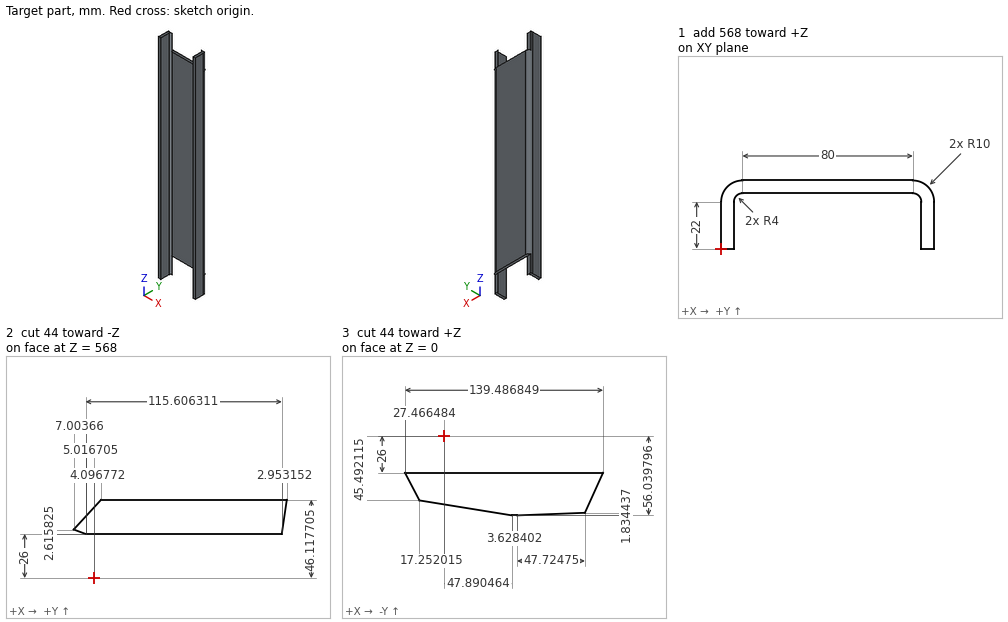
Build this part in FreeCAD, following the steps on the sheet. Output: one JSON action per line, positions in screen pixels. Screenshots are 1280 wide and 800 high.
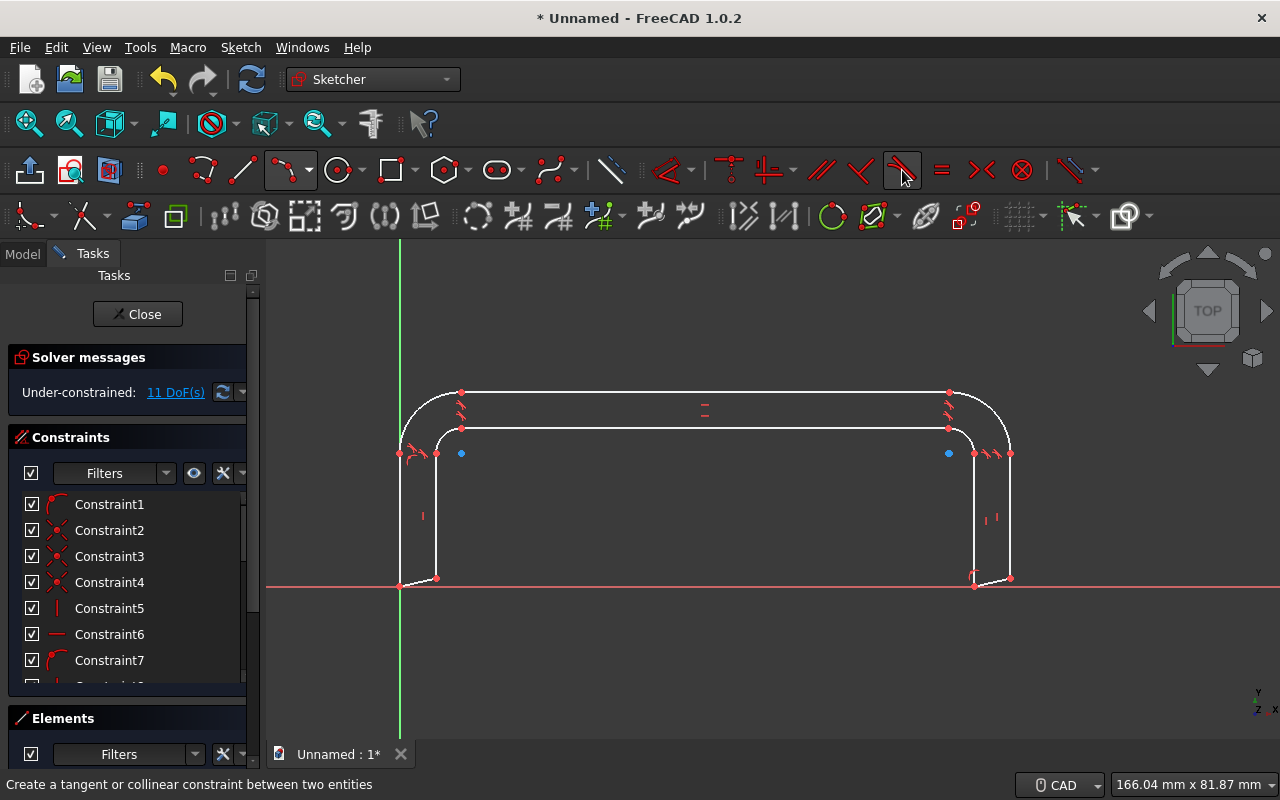
{"action": "scroll", "coordinate": [411, 584], "scroll_direction": "up", "scroll_amount": 2}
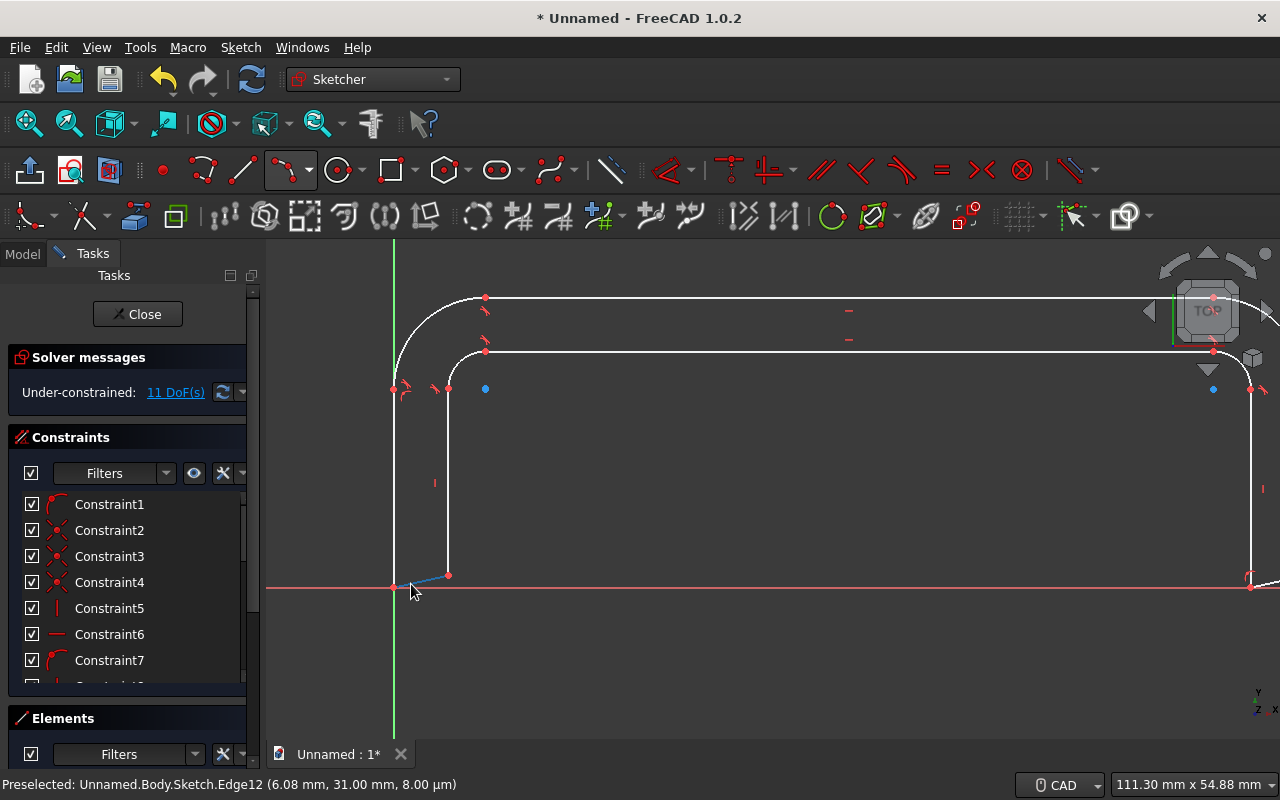
{"action": "left_click", "coordinate": [410, 584]}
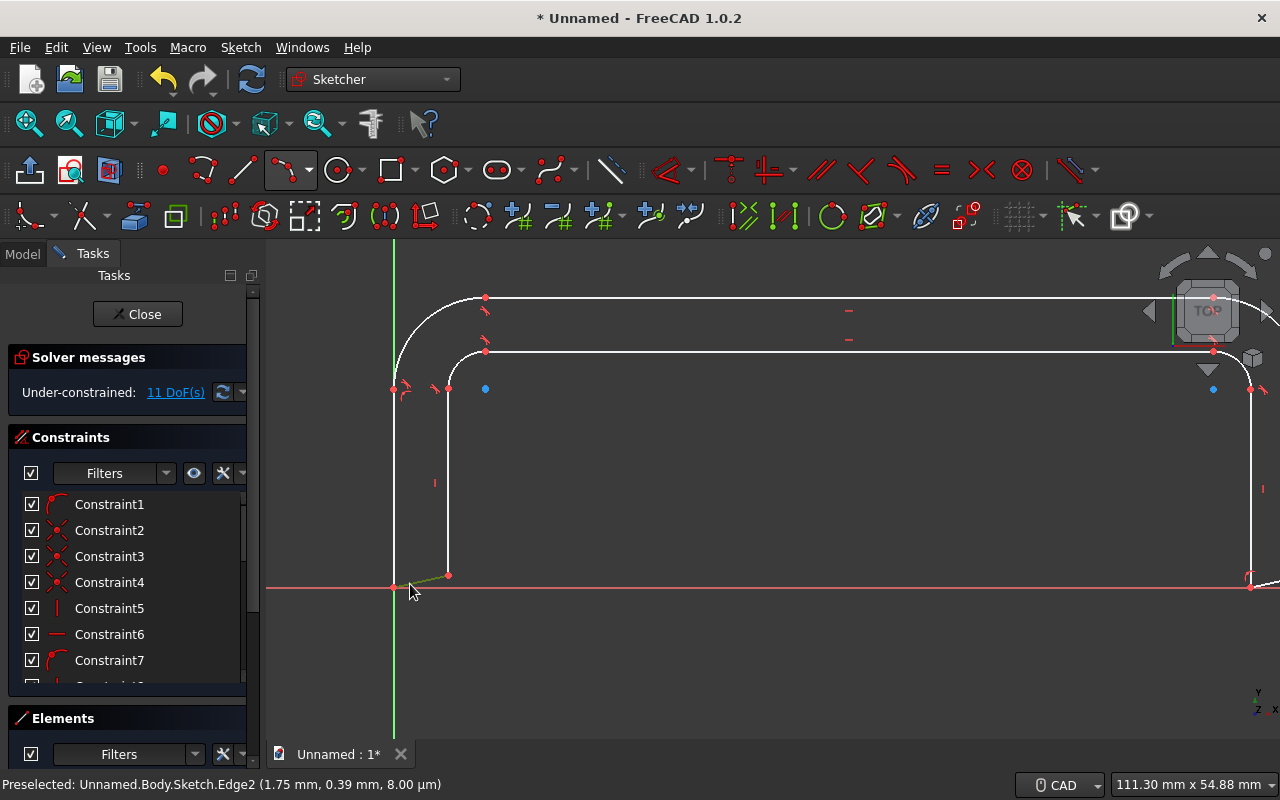
{"action": "left_click", "coordinate": [796, 170]}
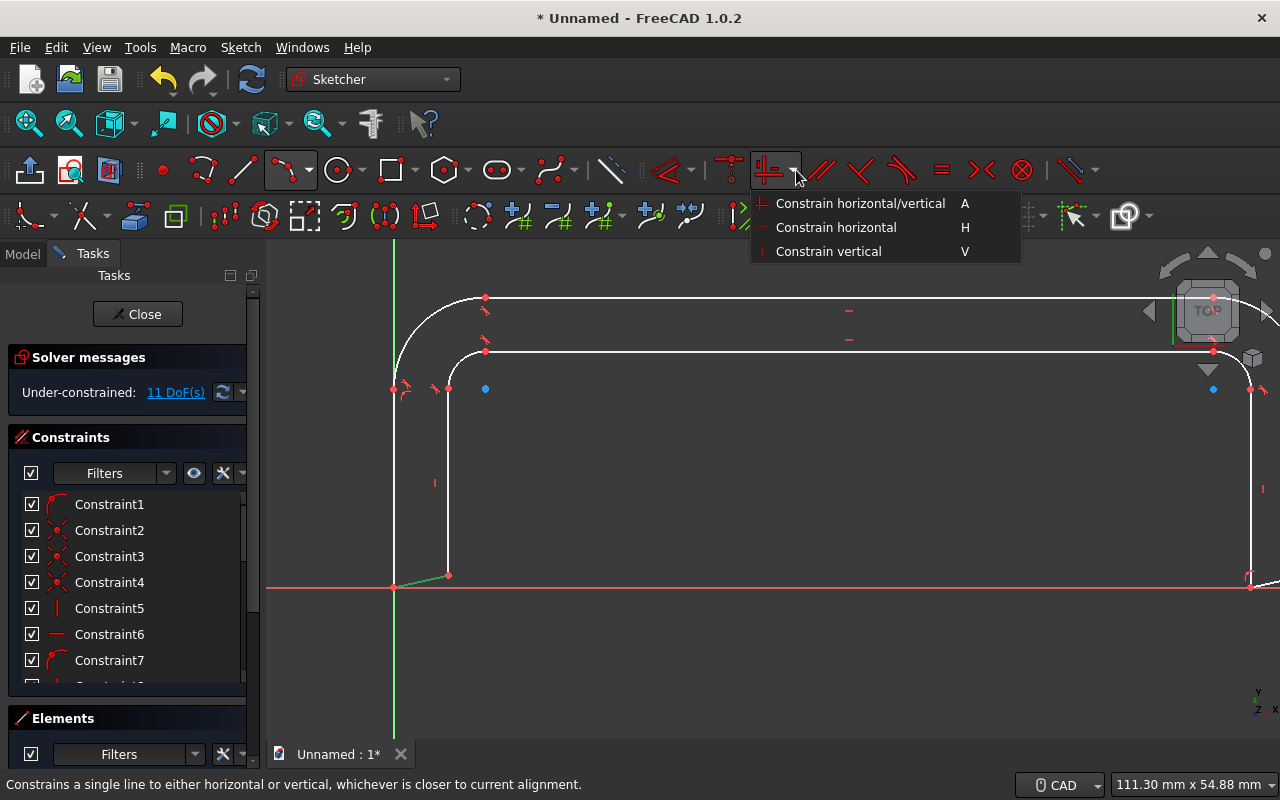
{"action": "left_click", "coordinate": [886, 227]}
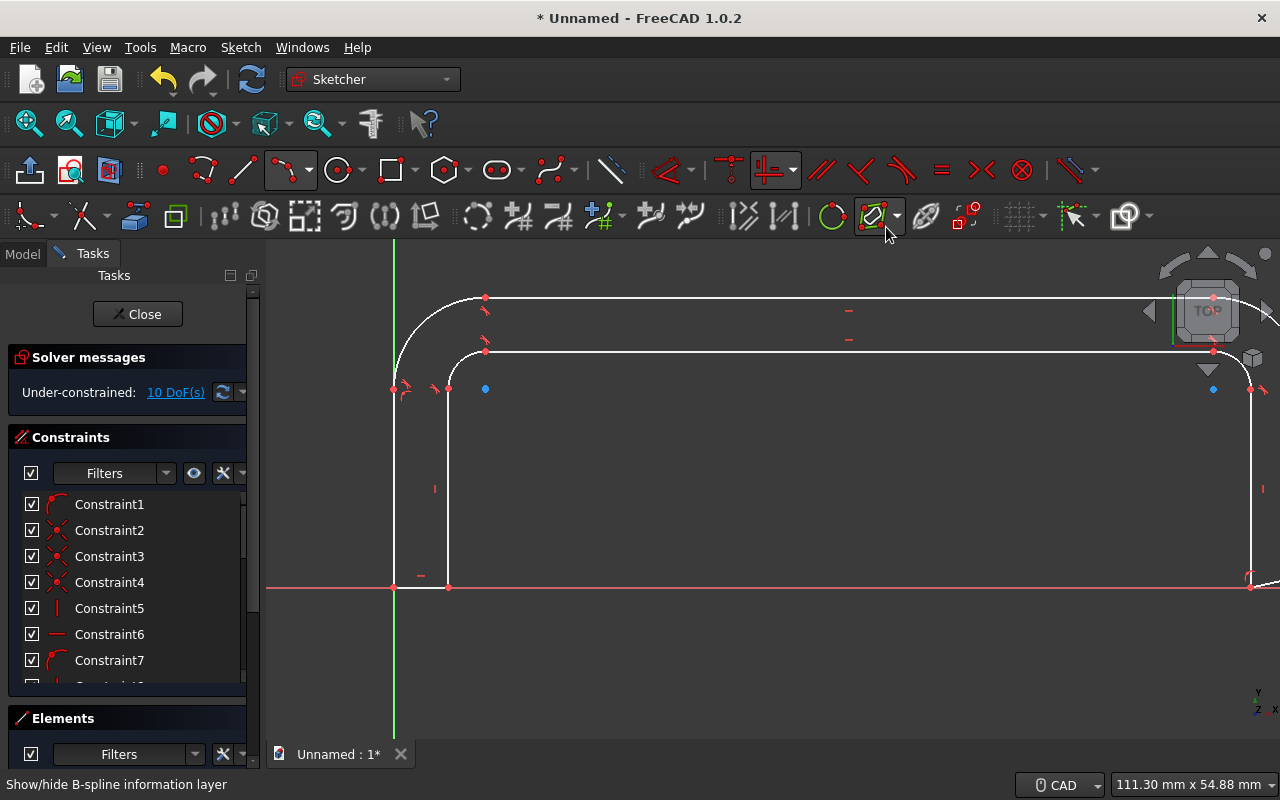
{"action": "scroll", "coordinate": [410, 585], "scroll_direction": "down", "scroll_amount": 2}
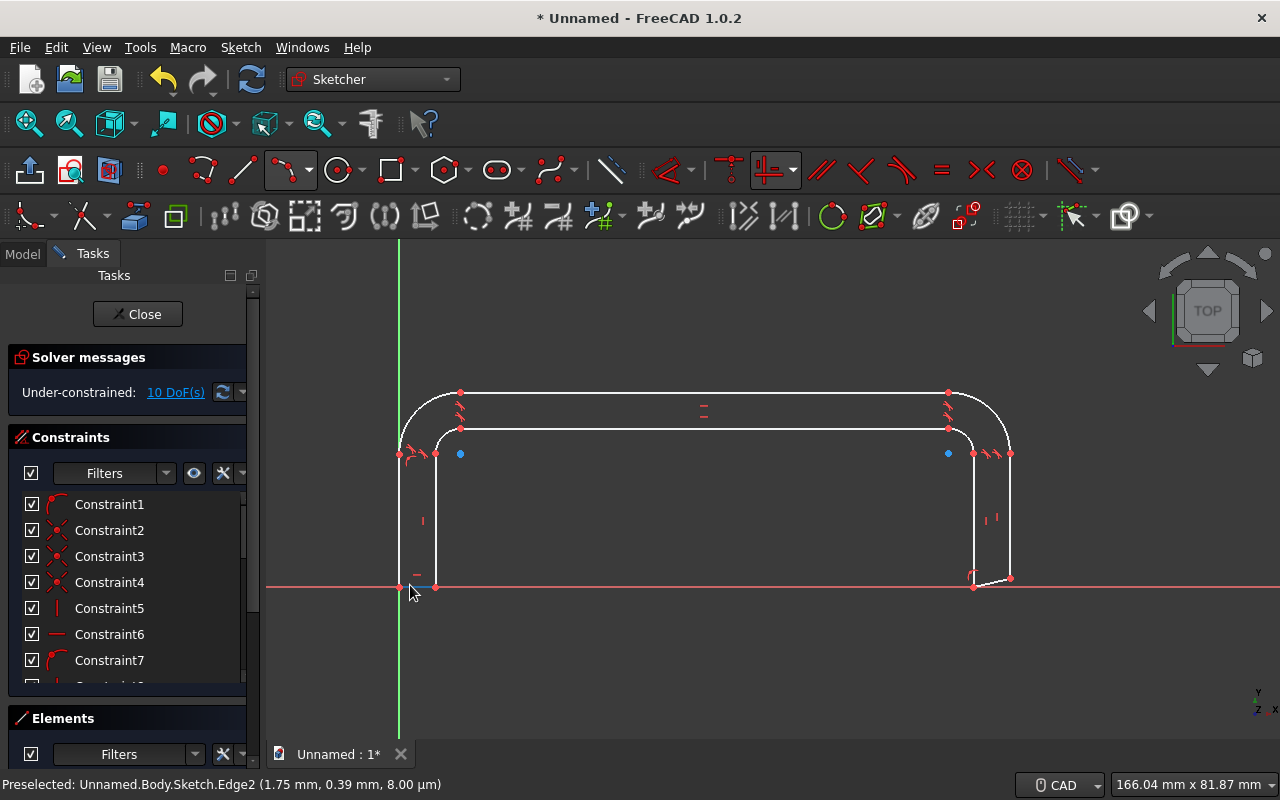
{"action": "scroll", "coordinate": [985, 585], "scroll_direction": "up", "scroll_amount": 2}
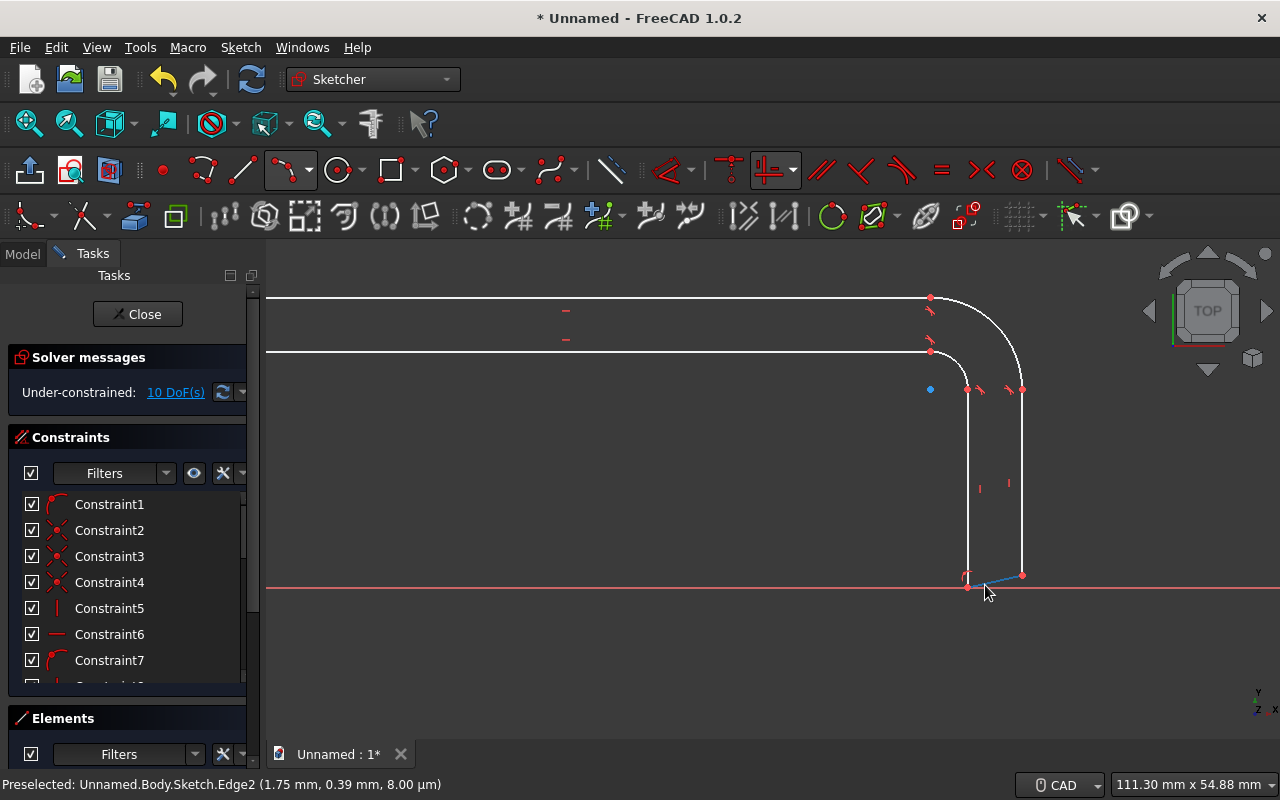
{"action": "left_click", "coordinate": [984, 584]}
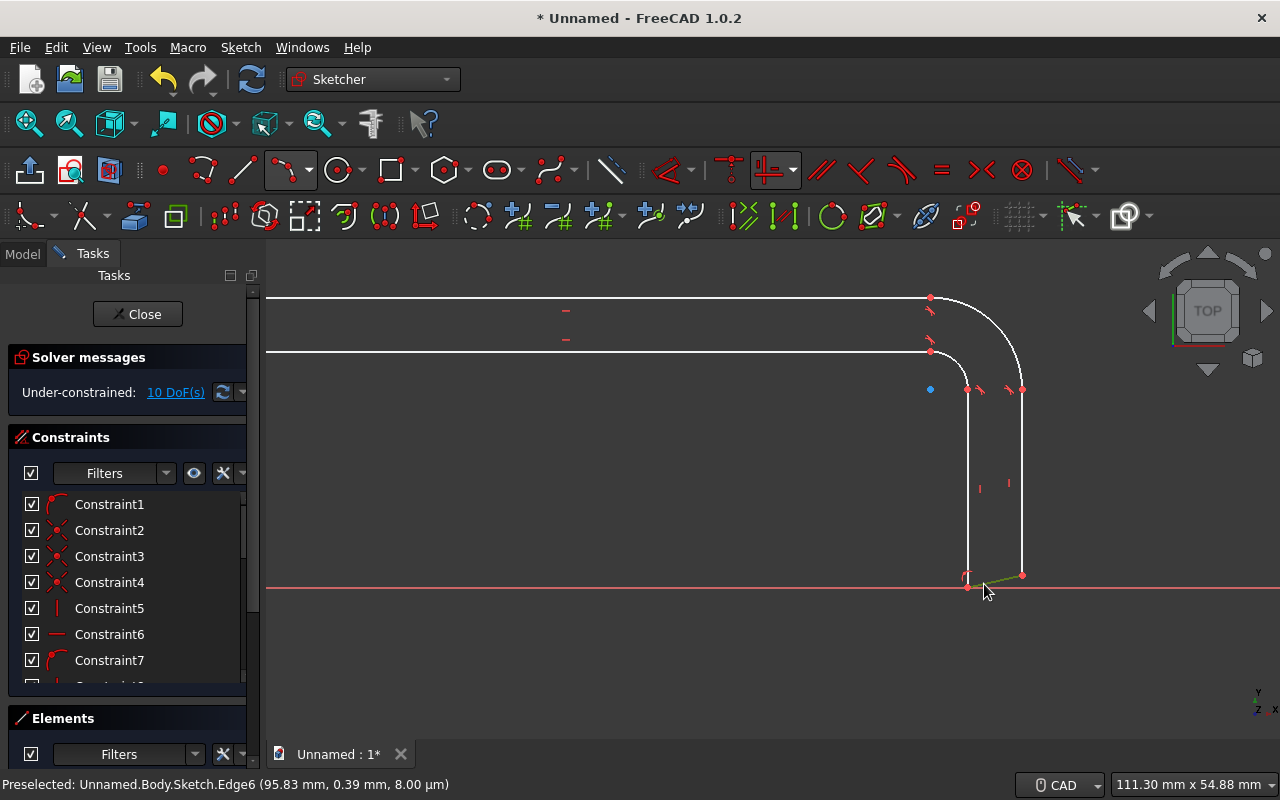
{"action": "key", "text": "h"}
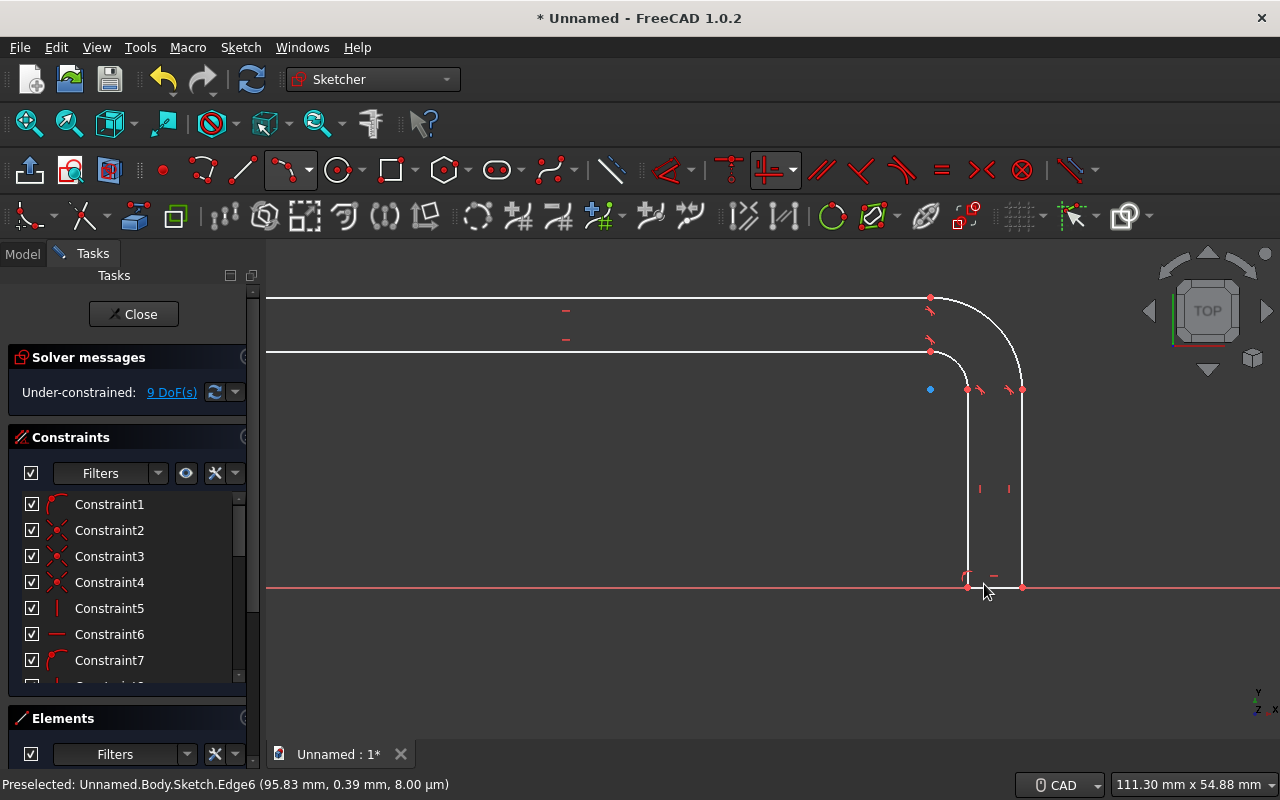
{"action": "left_click", "coordinate": [964, 372]}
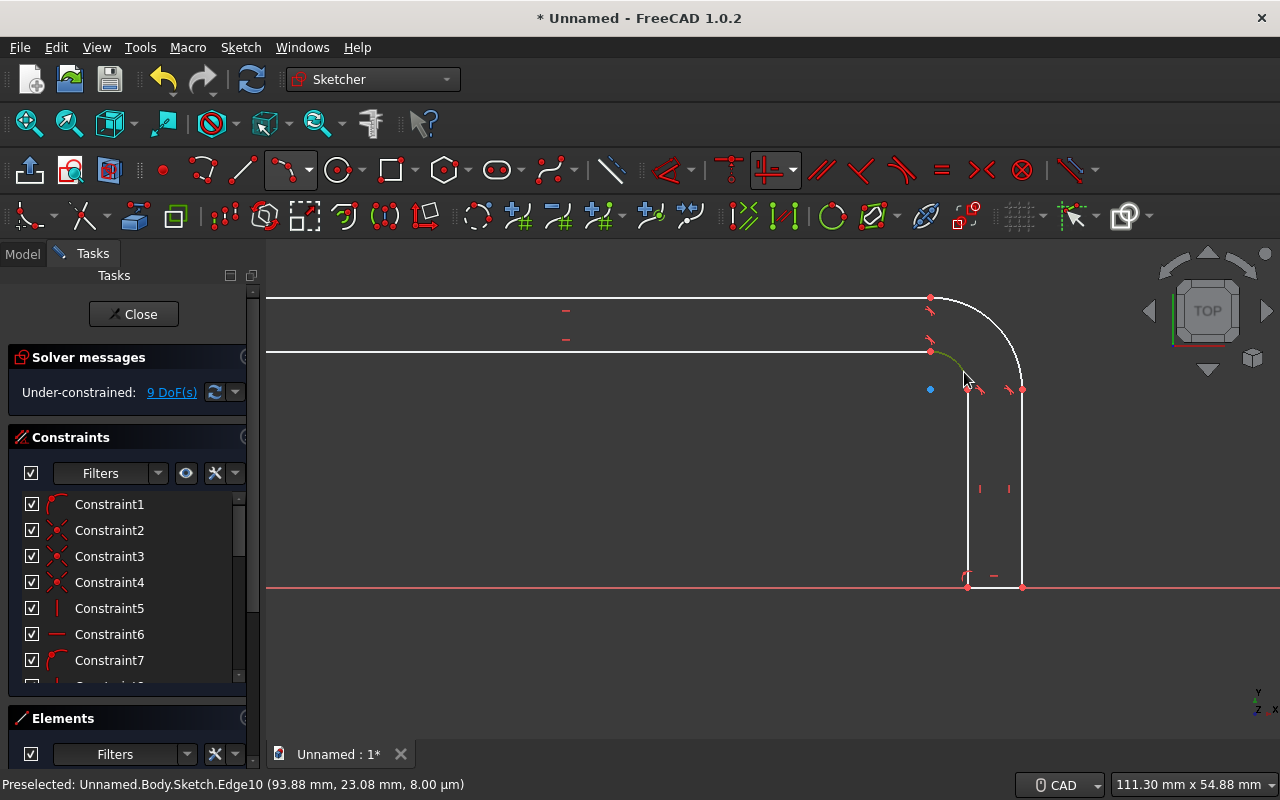
{"action": "left_click", "coordinate": [1012, 348]}